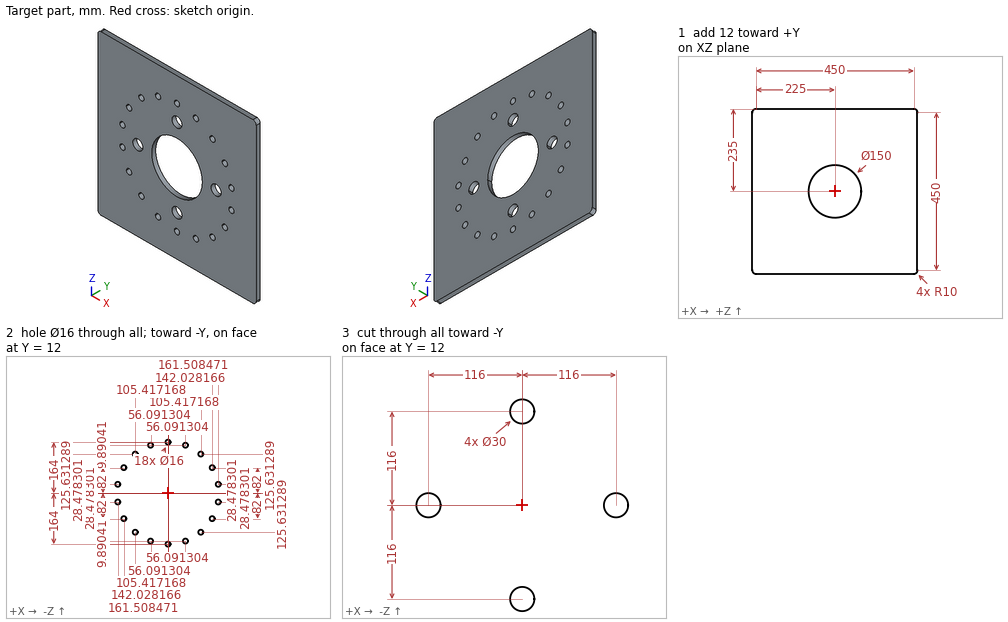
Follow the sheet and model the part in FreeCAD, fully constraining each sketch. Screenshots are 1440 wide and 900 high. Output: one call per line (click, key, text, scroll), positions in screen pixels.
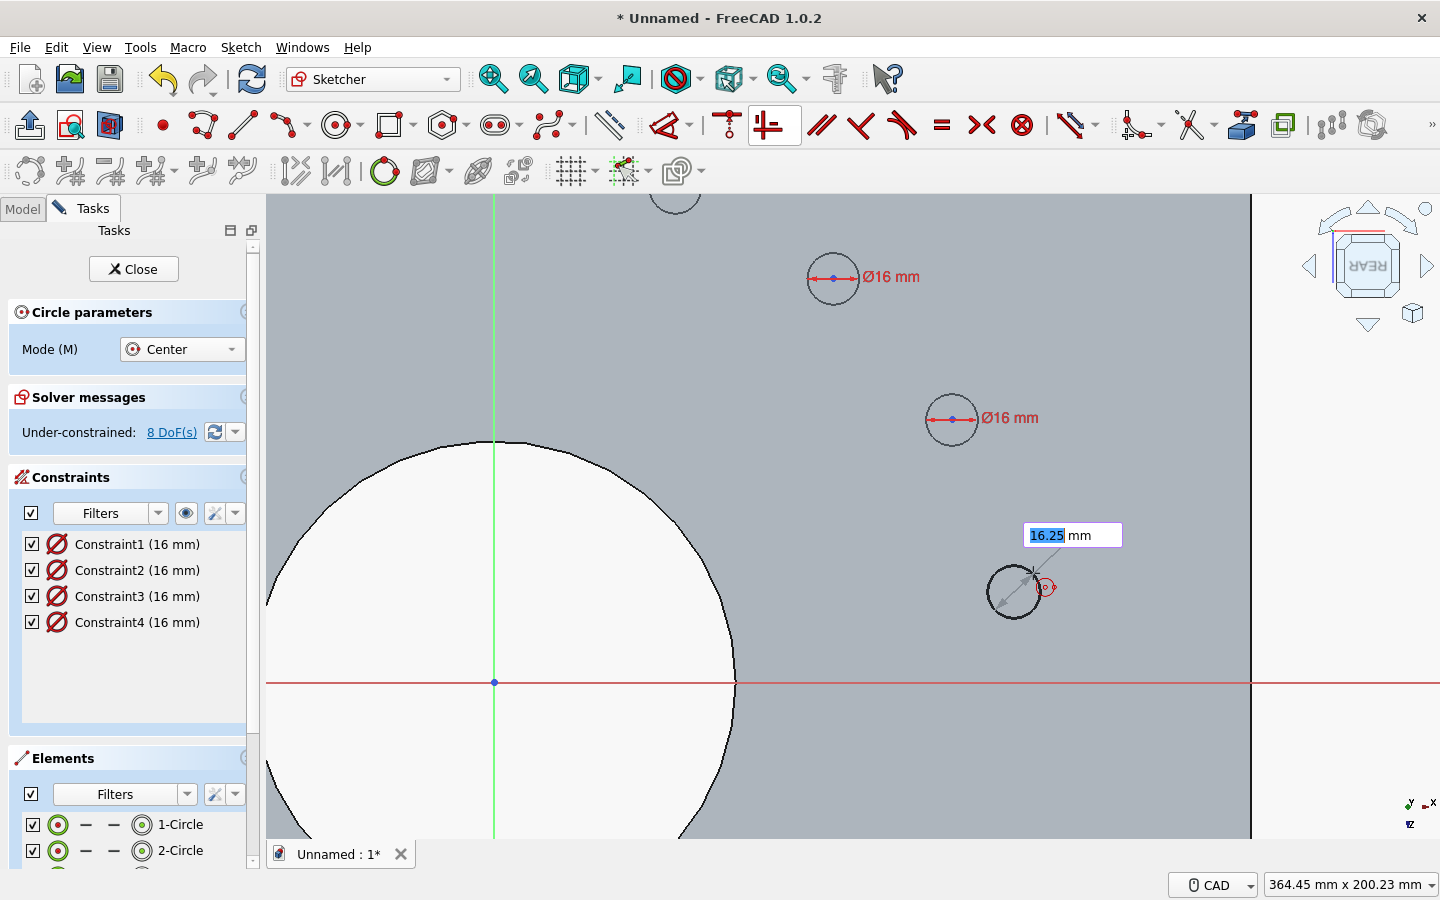
text(16)
key(Return)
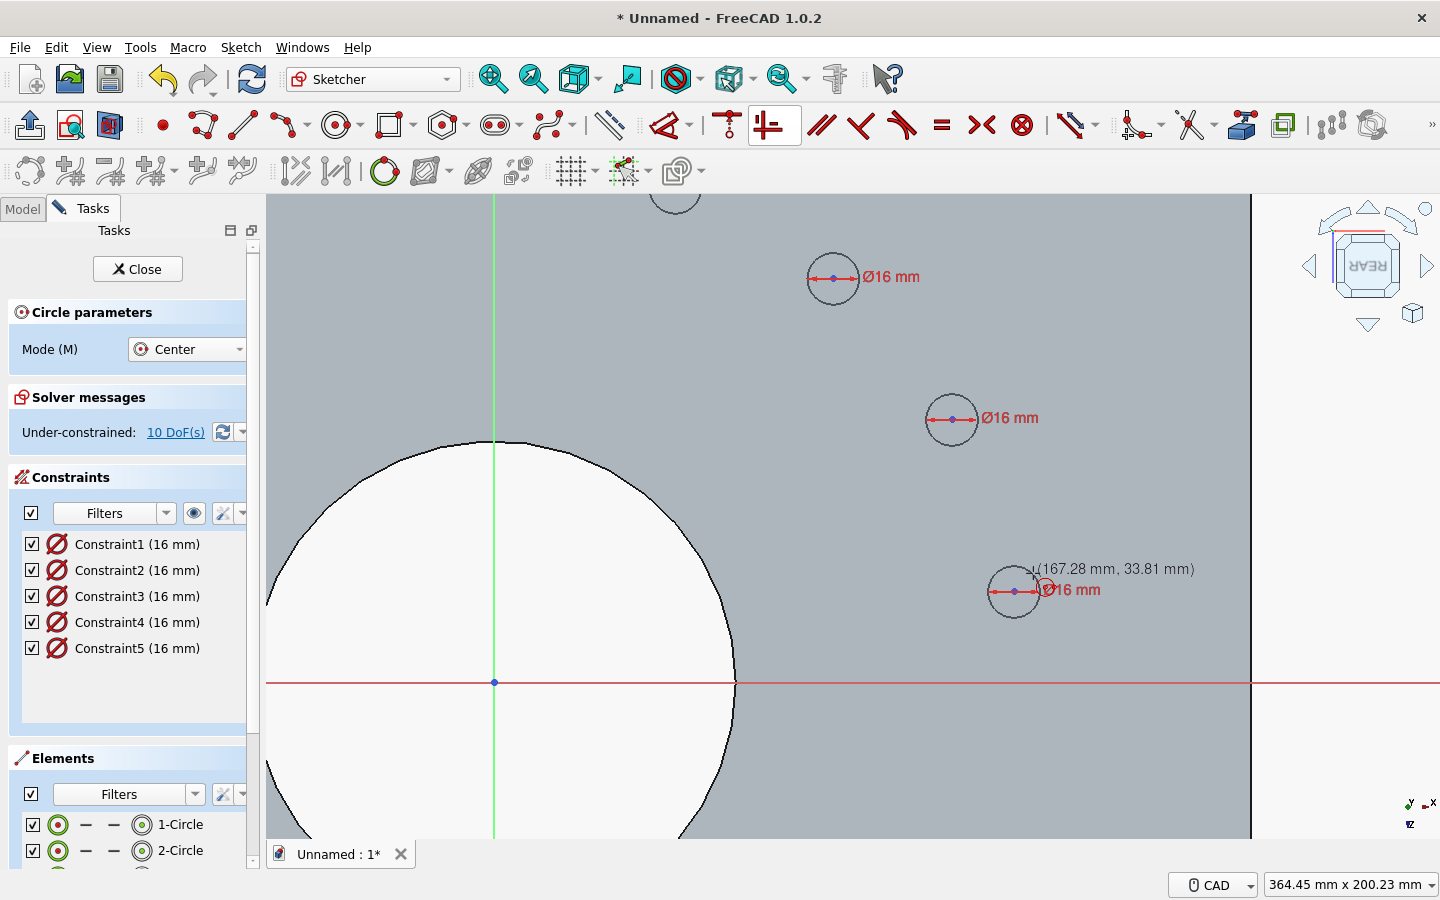
click(1014, 775)
move(1033, 756)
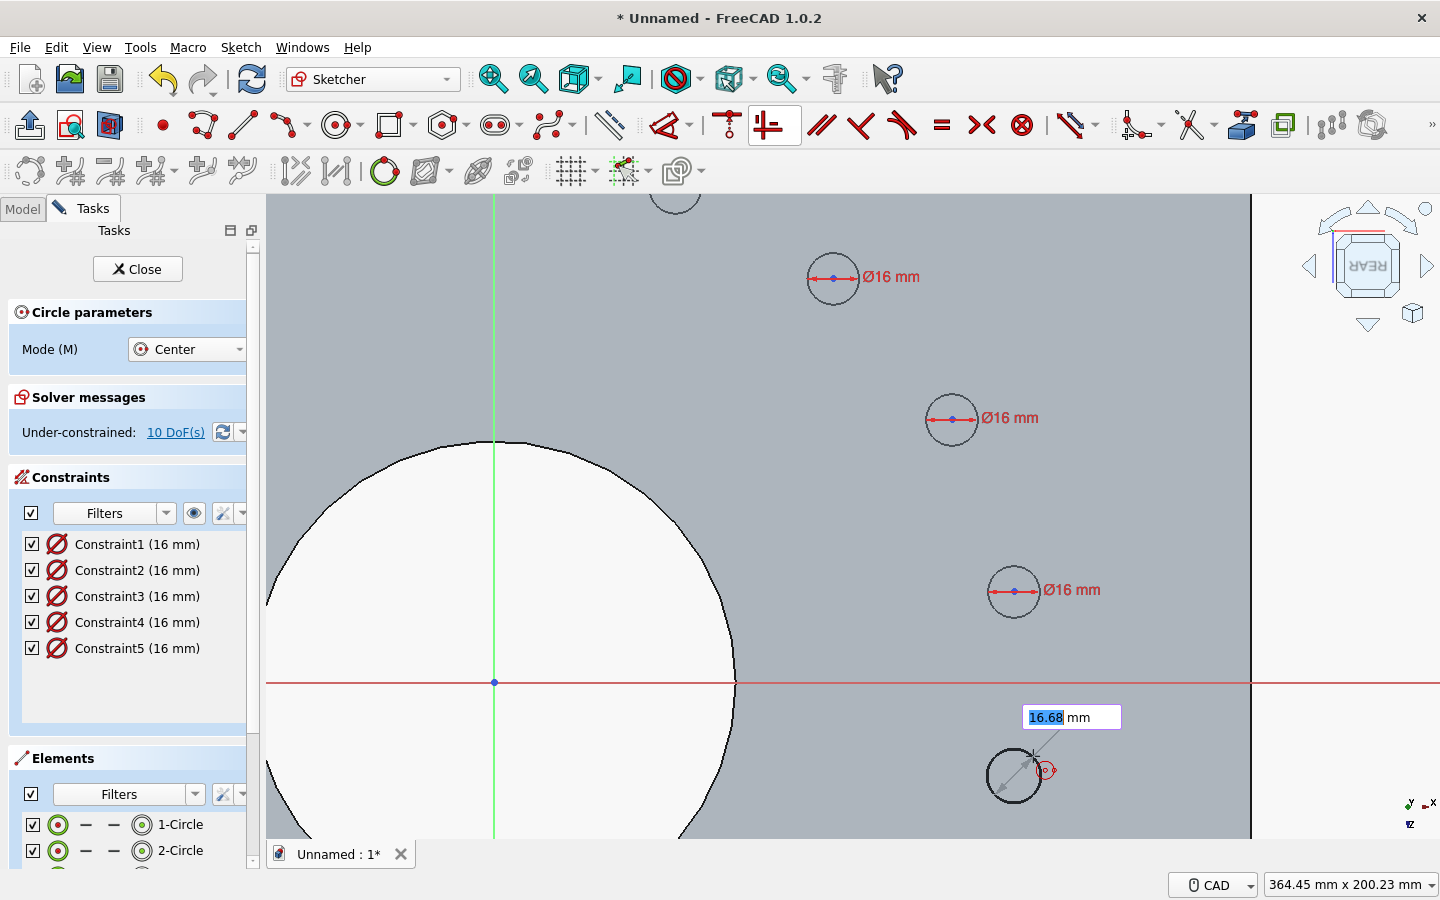
text(16)
key(Return)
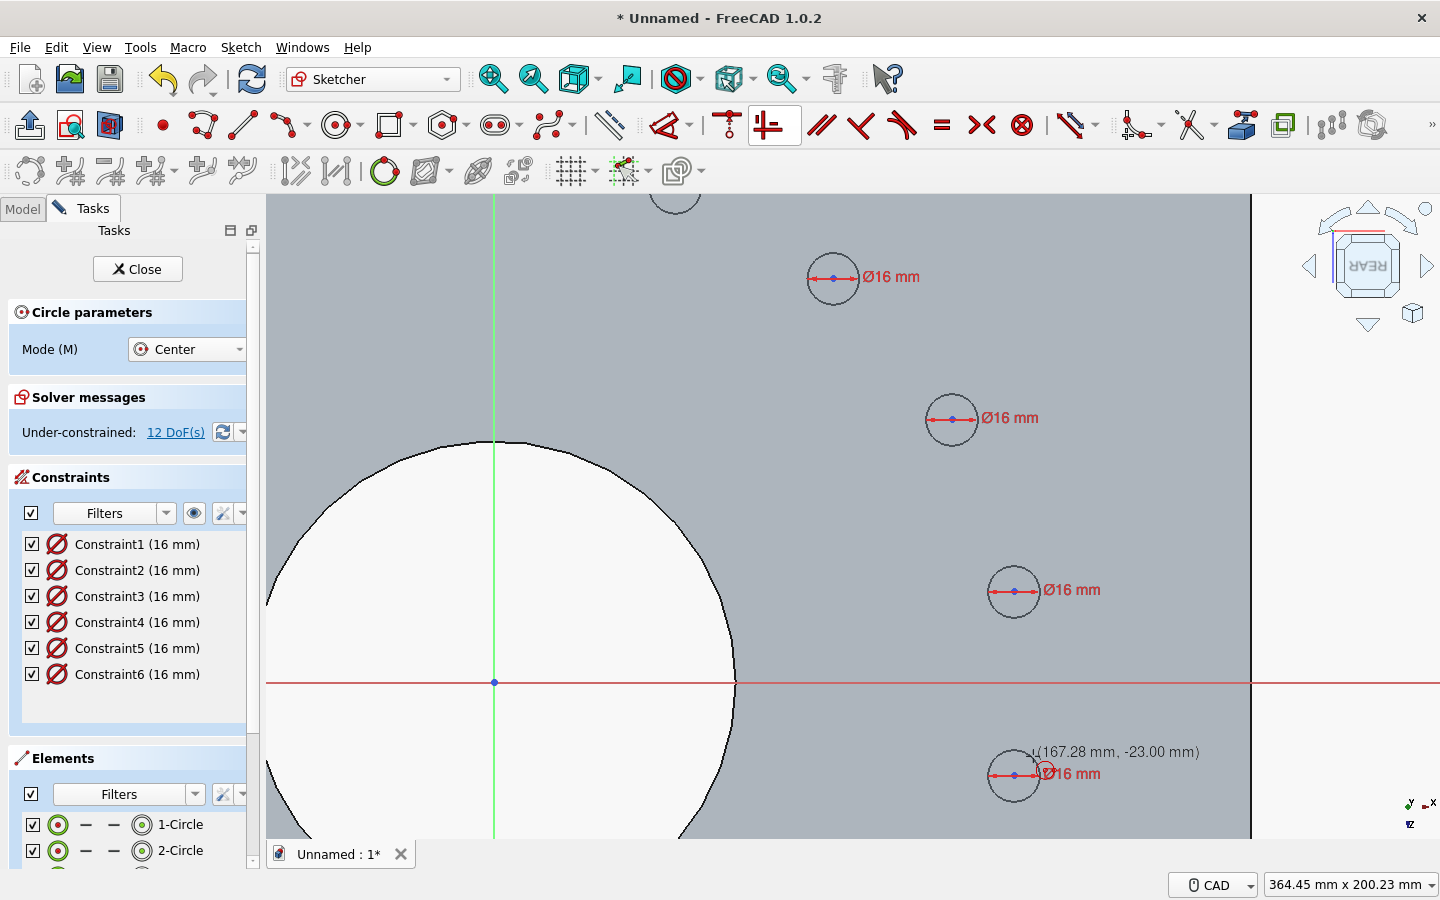
scroll(953, 420, down, 5)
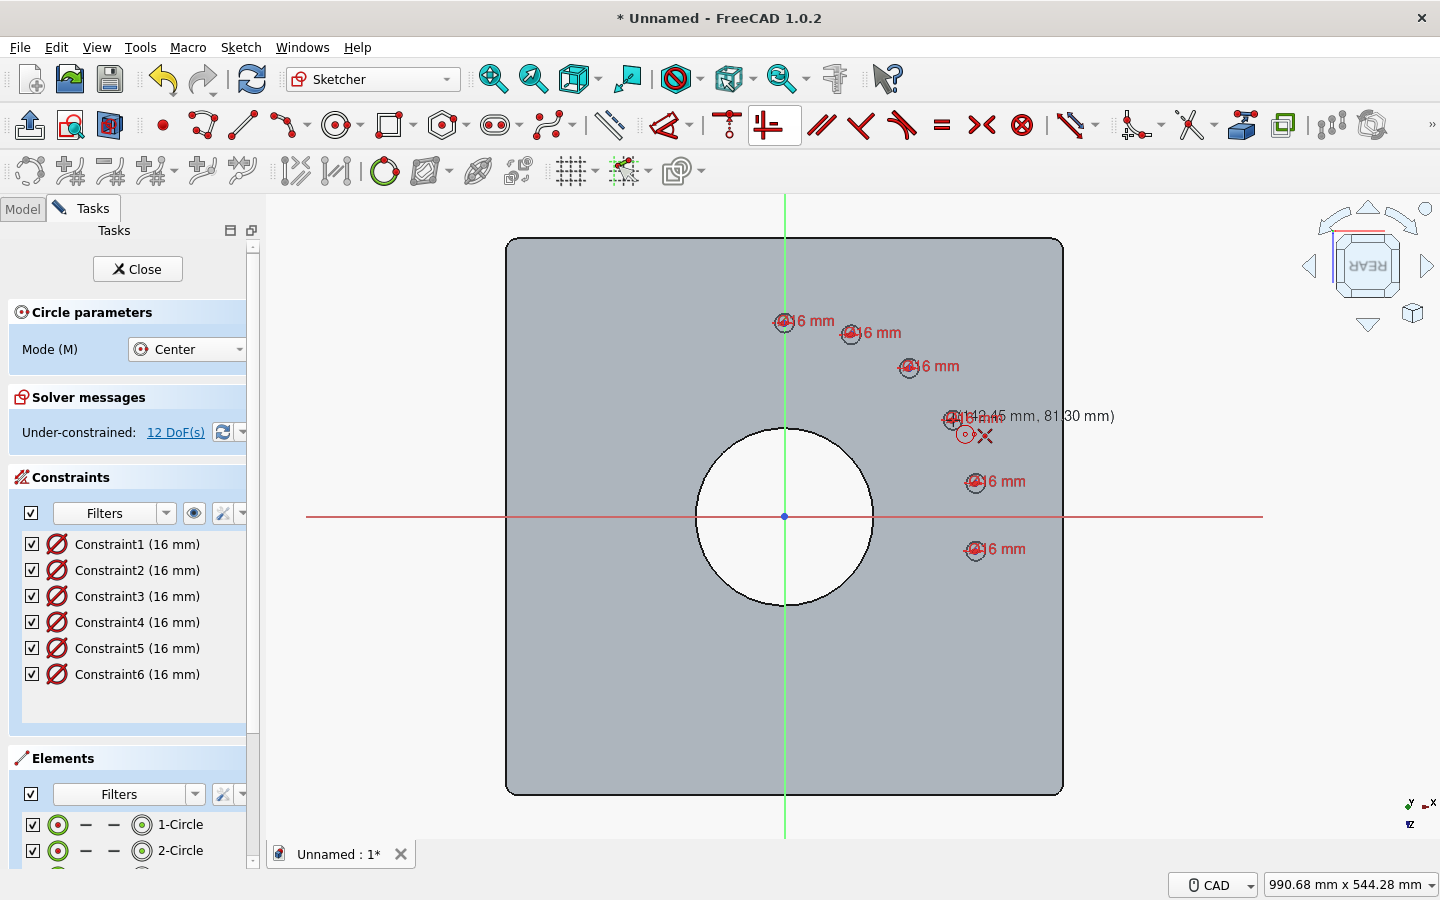
scroll(953, 614, up, 5)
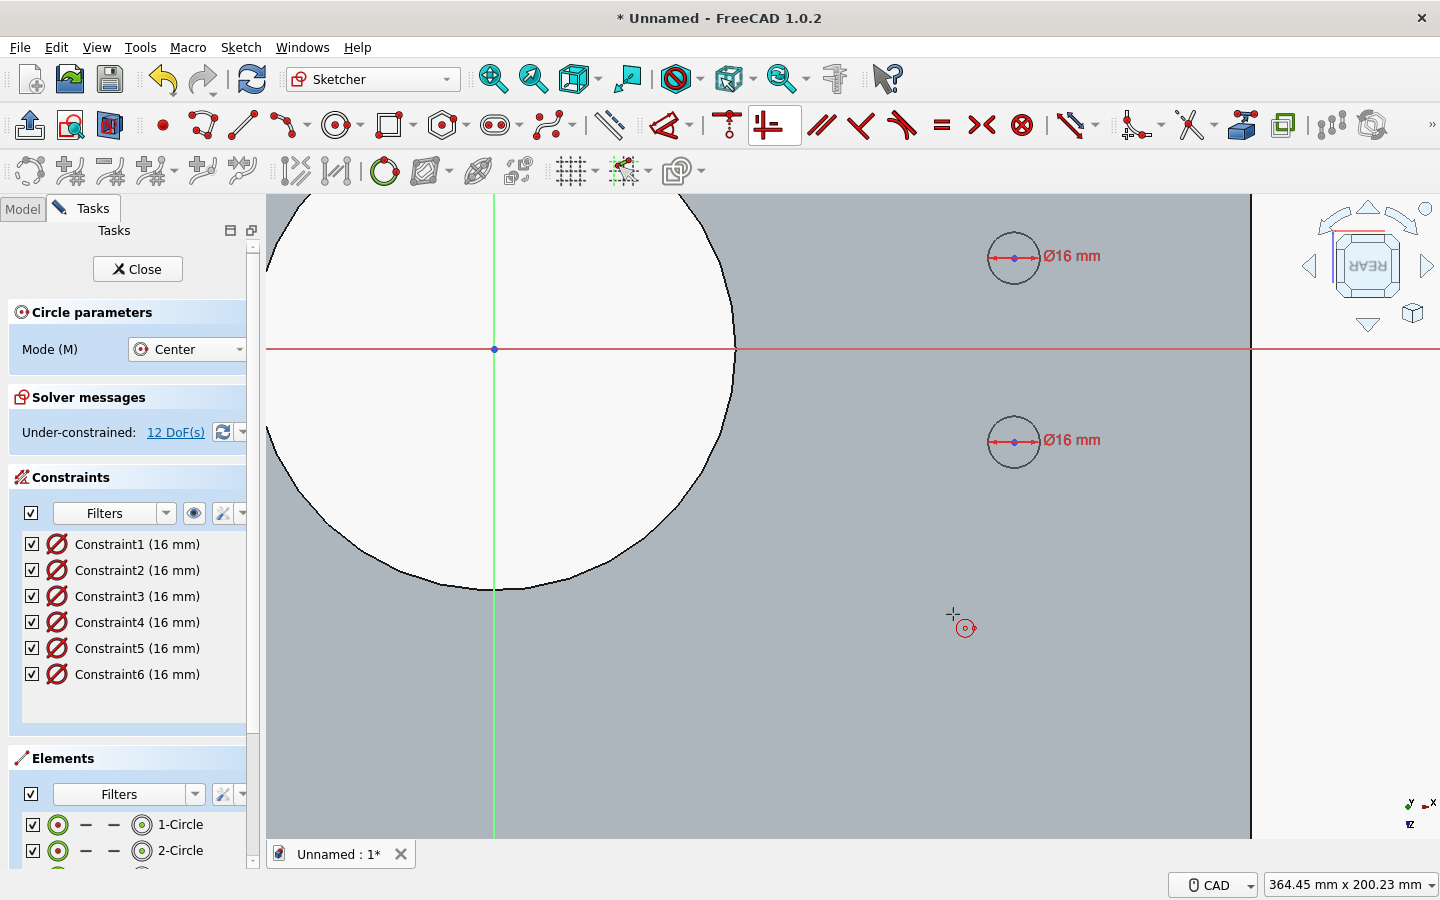
click(952, 613)
move(970, 595)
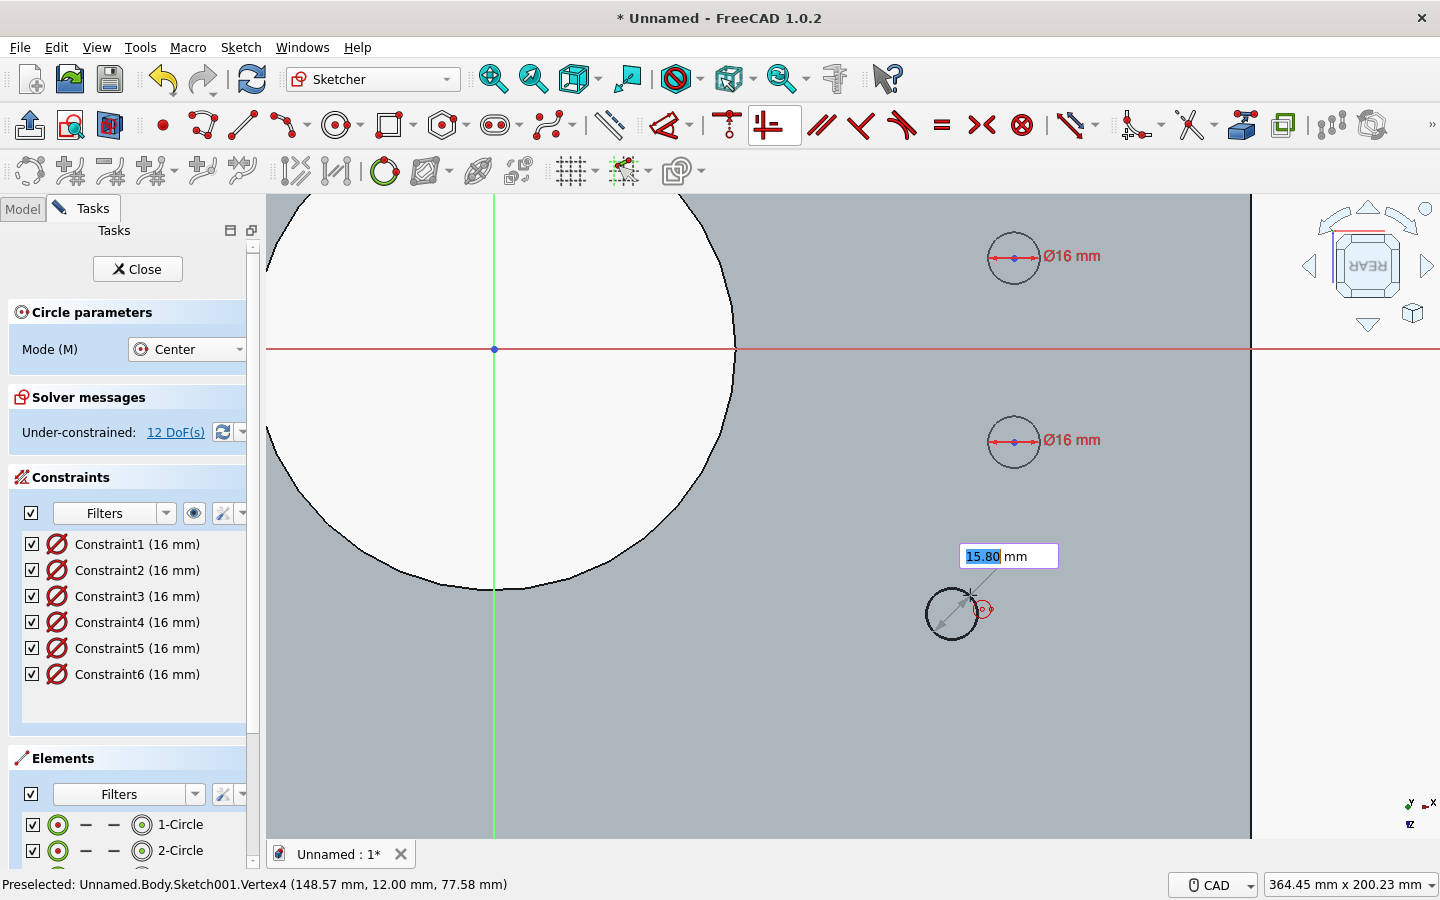
text(16)
key(Return)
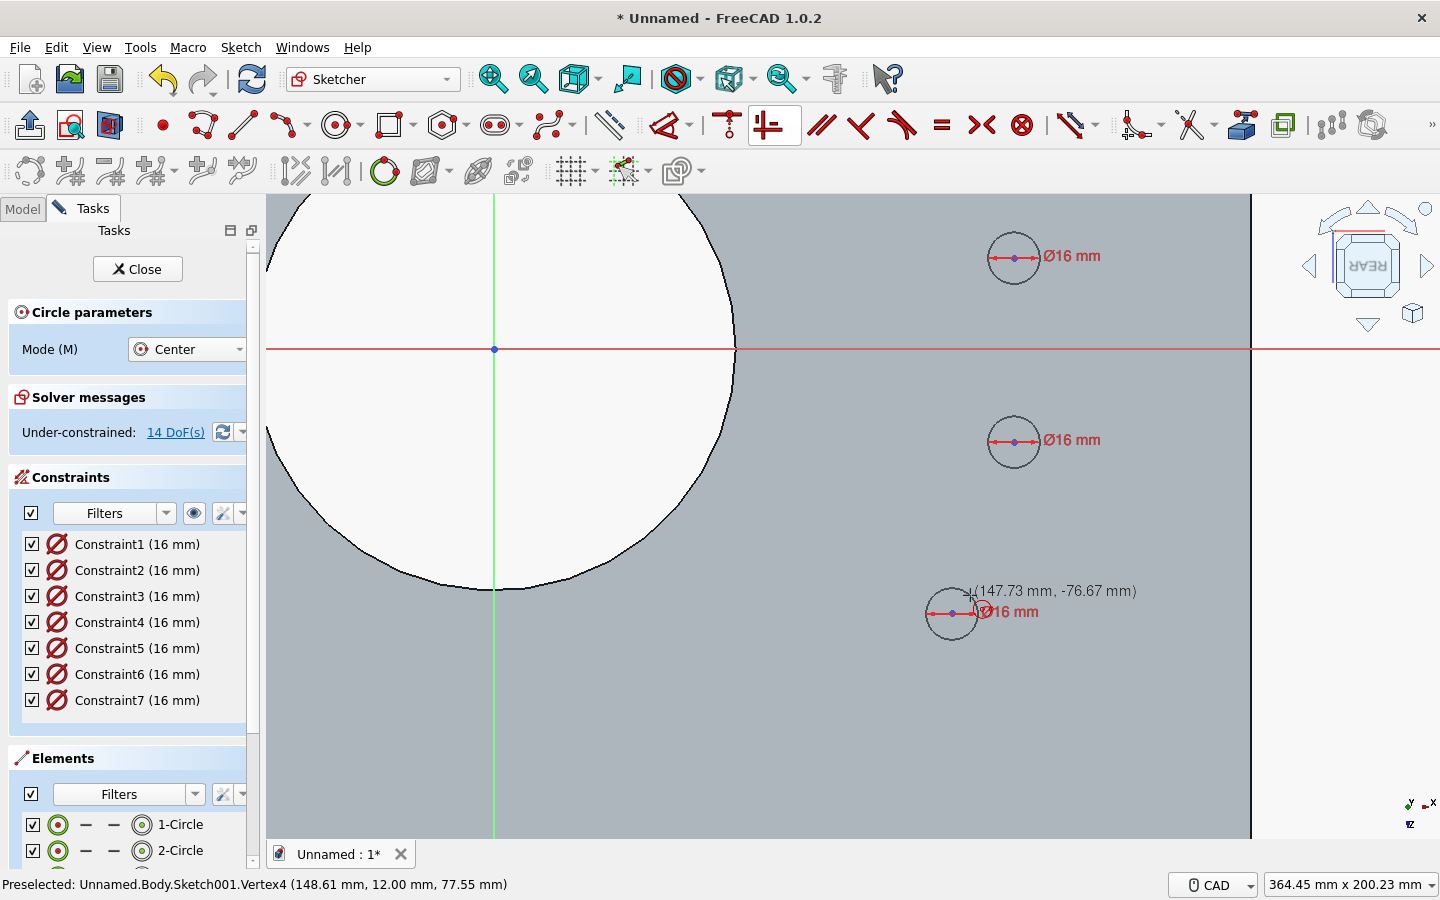
click(834, 754)
move(852, 736)